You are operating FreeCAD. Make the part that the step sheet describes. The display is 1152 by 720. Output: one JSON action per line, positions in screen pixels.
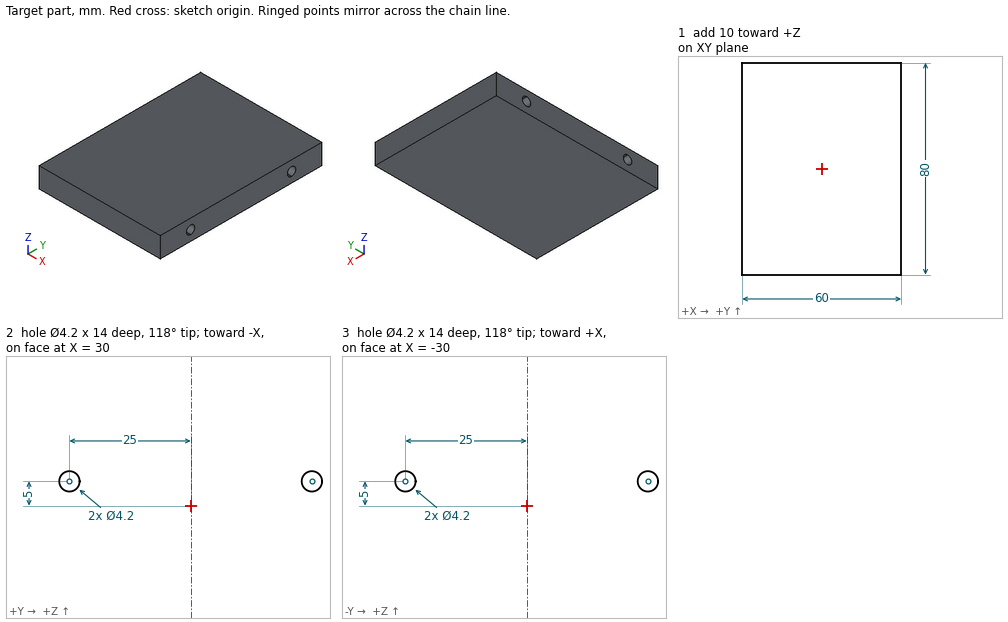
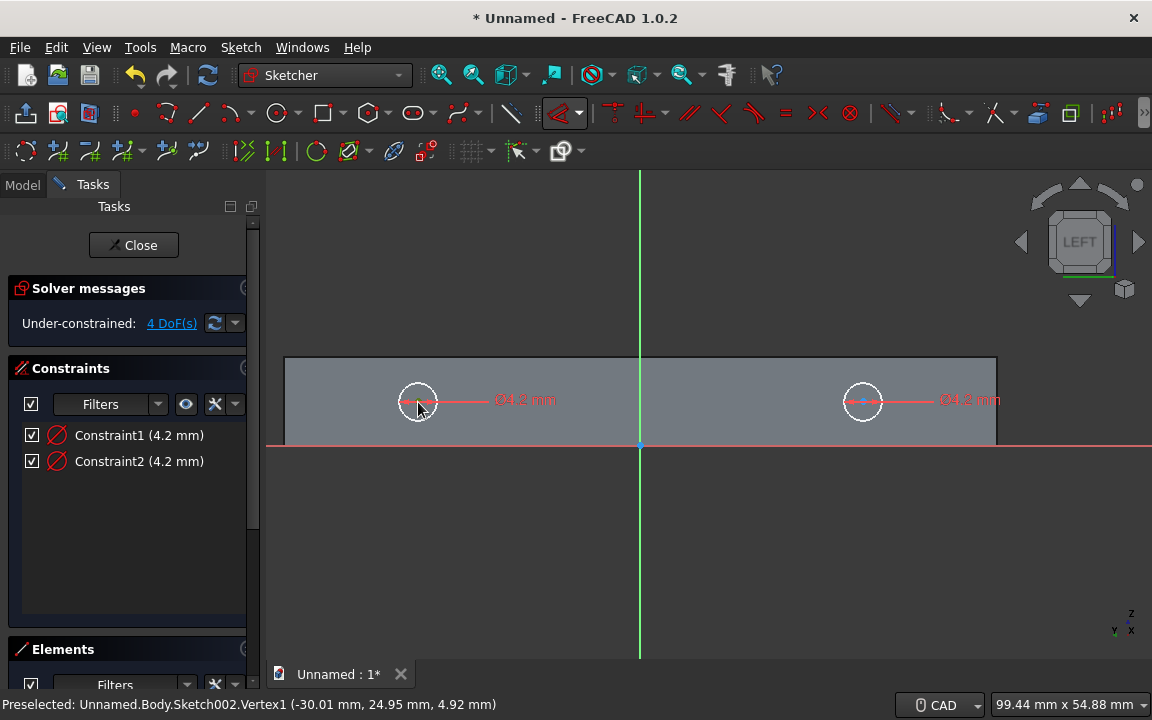
{"action": "left_click", "coordinate": [863, 402]}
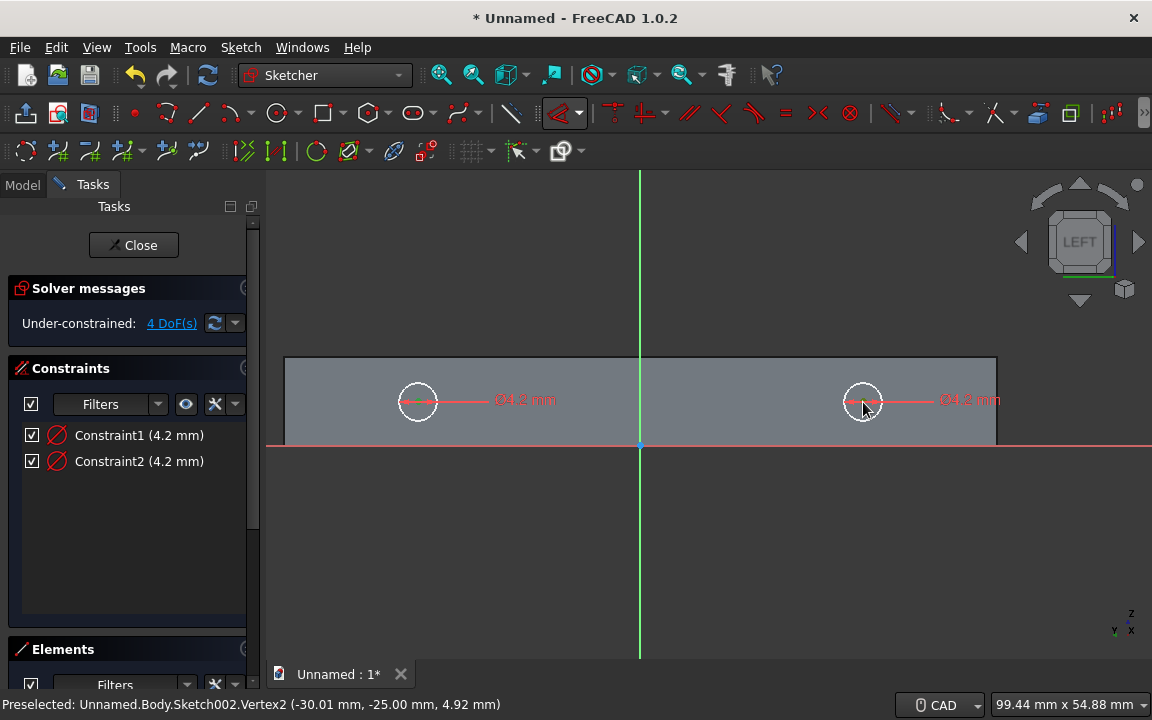
{"action": "left_click", "coordinate": [640, 600]}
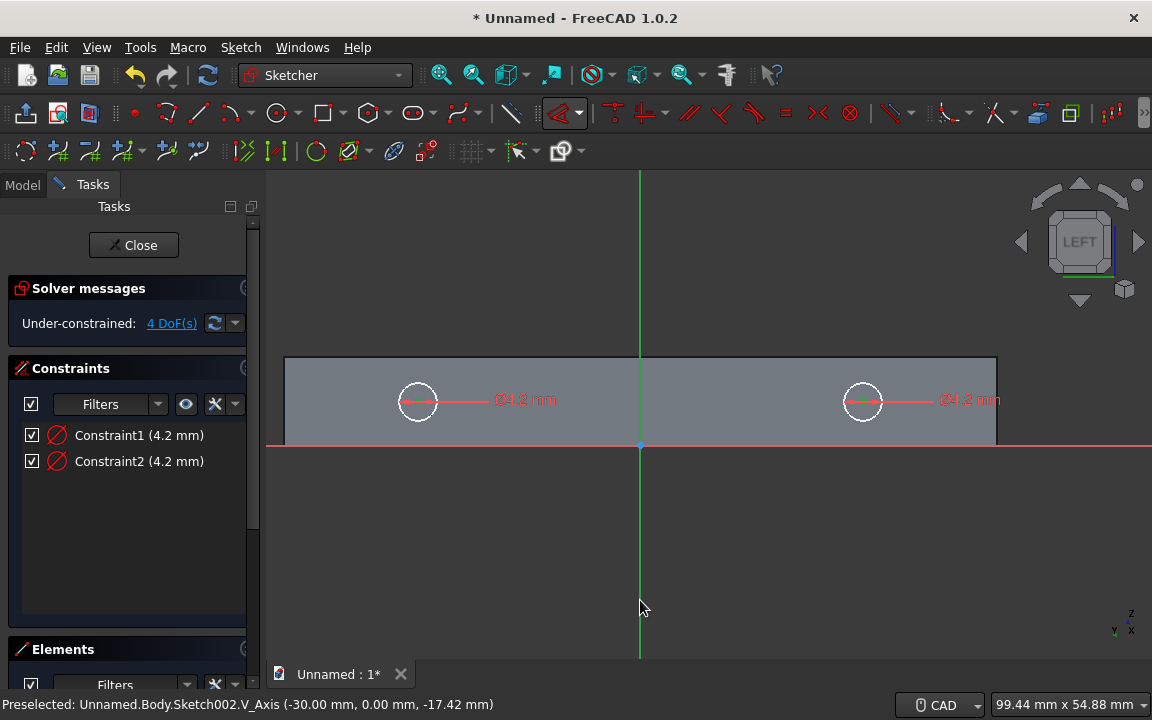
{"action": "left_click", "coordinate": [818, 114]}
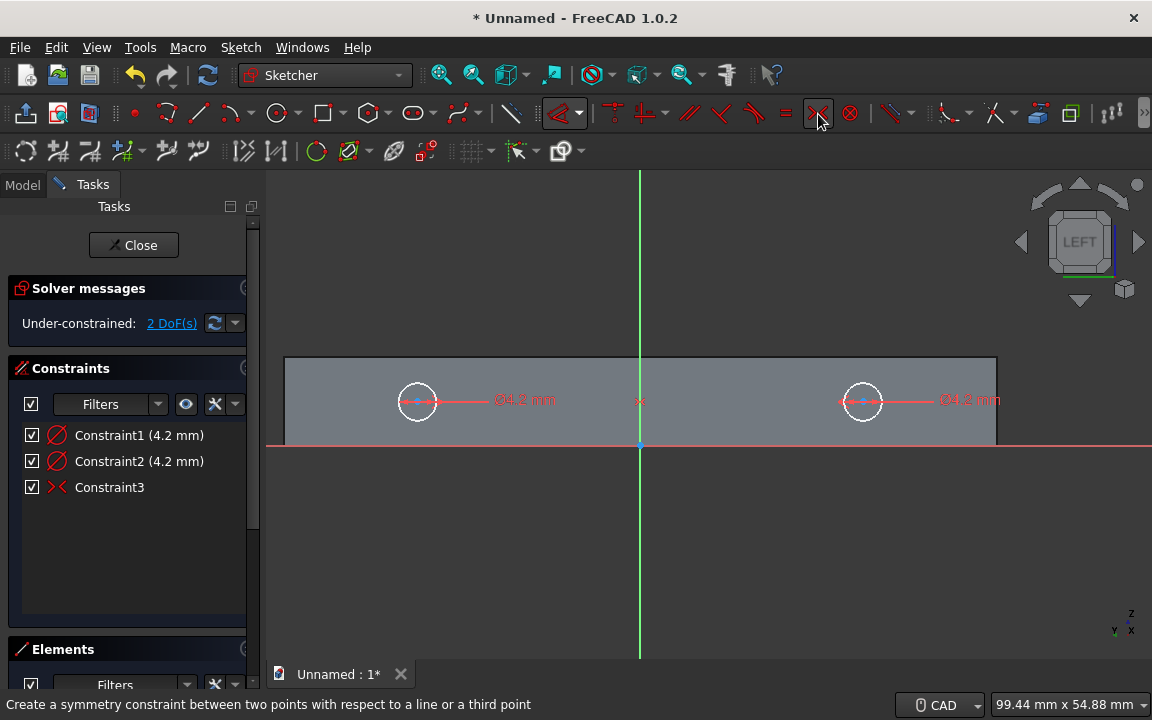
{"action": "left_click", "coordinate": [418, 402]}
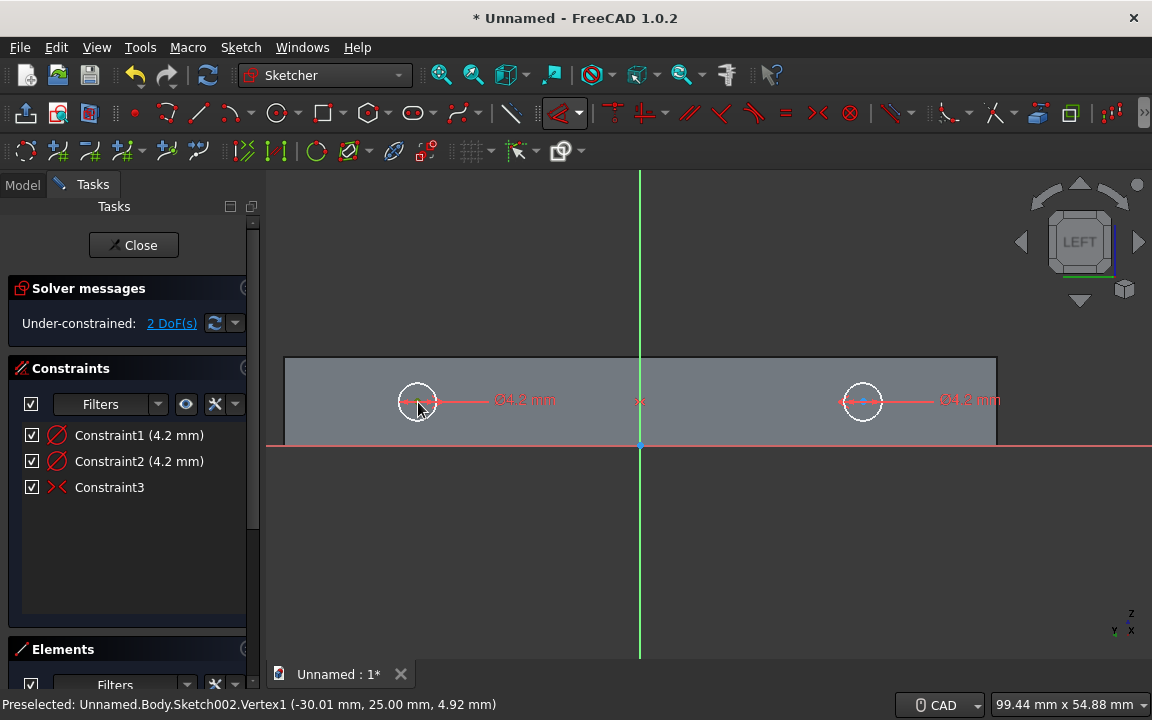
{"action": "left_click", "coordinate": [582, 114]}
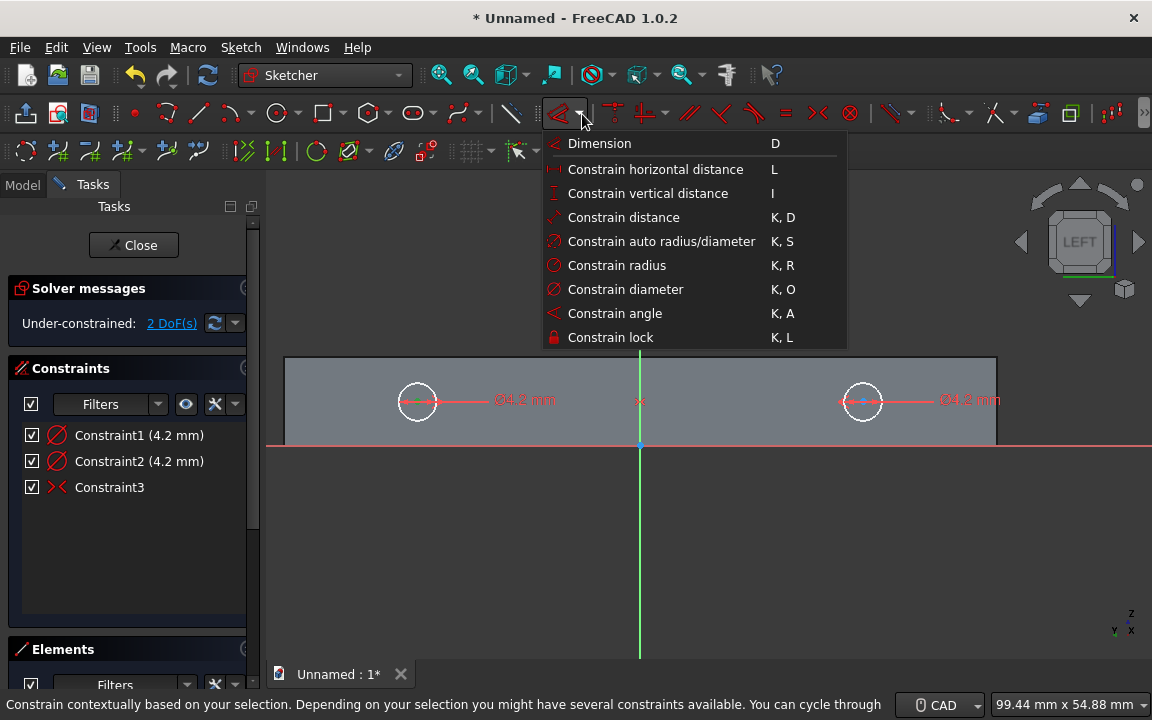
{"action": "left_click", "coordinate": [695, 193]}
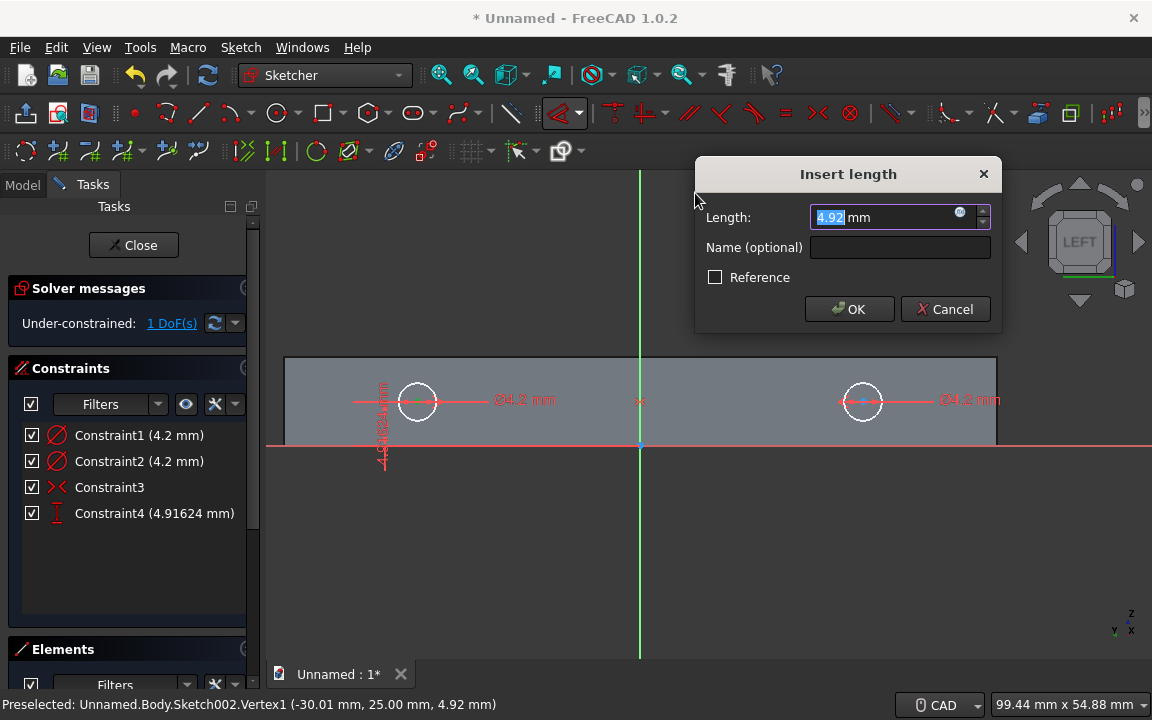
{"action": "type", "text": "5"}
{"action": "key", "text": "Return"}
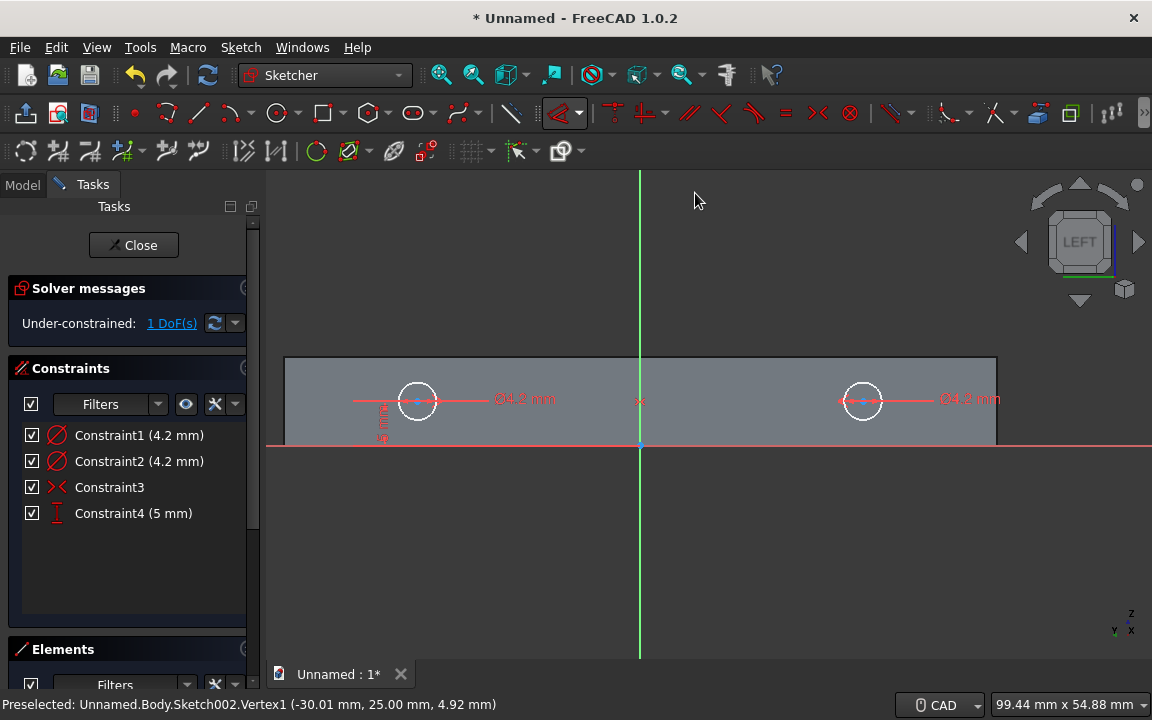
{"action": "left_click", "coordinate": [418, 401]}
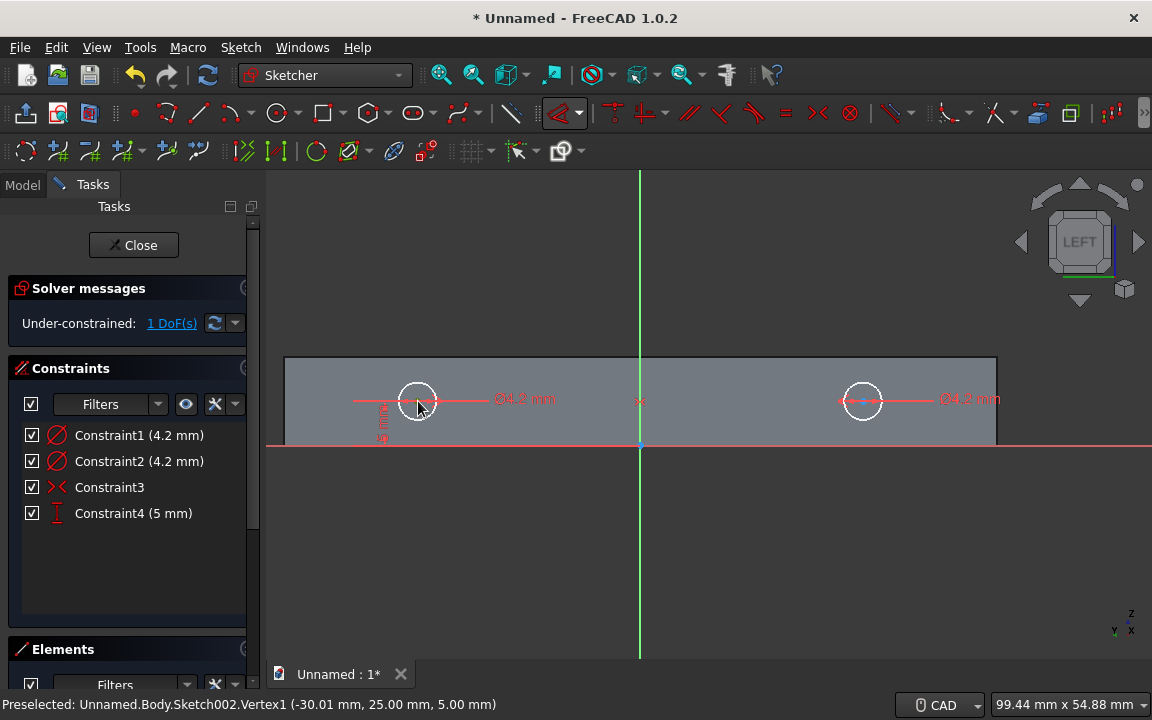
{"action": "left_click", "coordinate": [582, 114]}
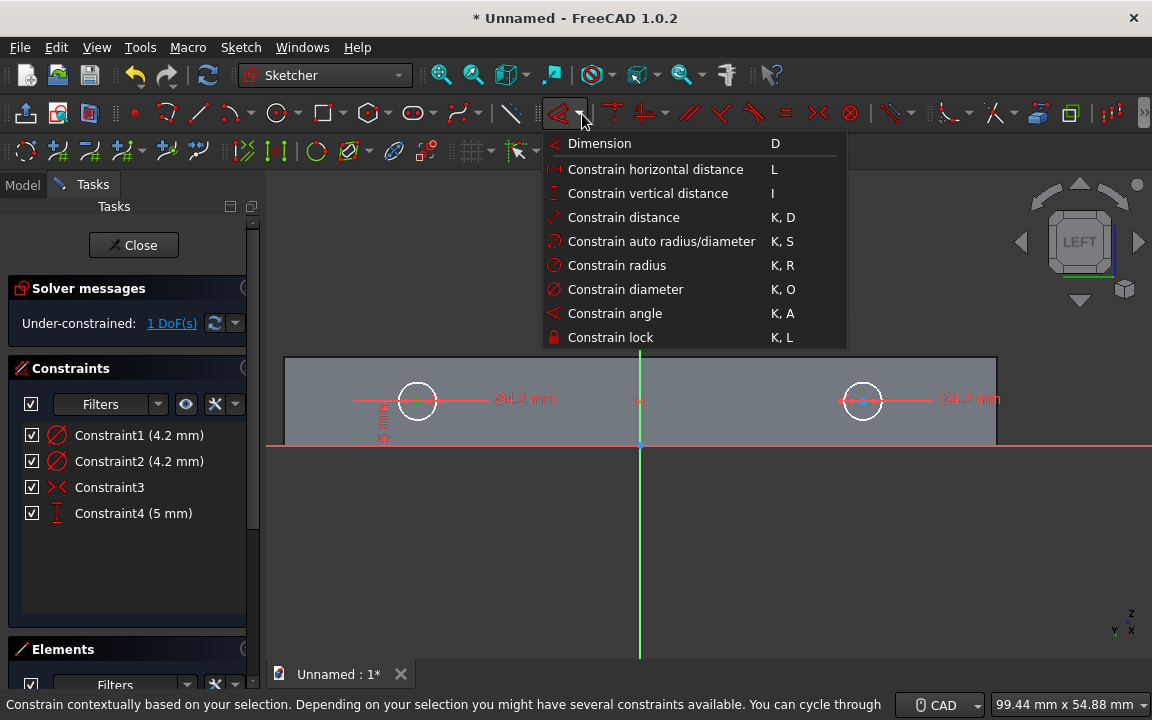
{"action": "left_click", "coordinate": [695, 169]}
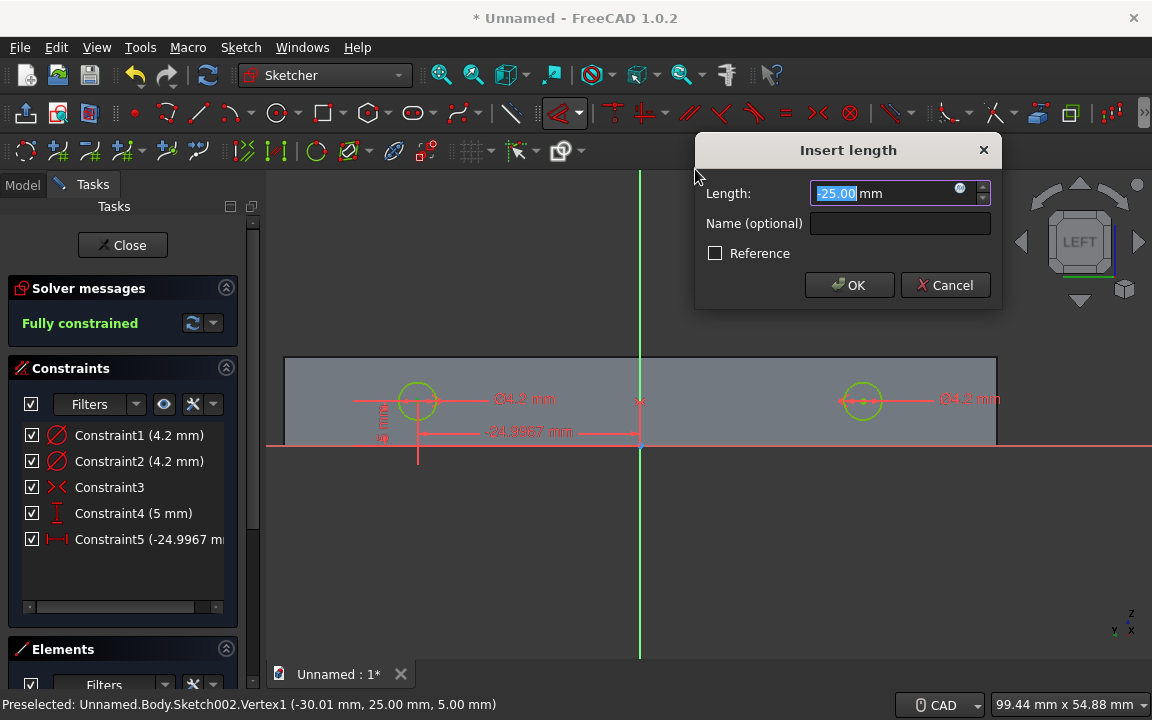
{"action": "type", "text": "-25"}
{"action": "key", "text": "Return"}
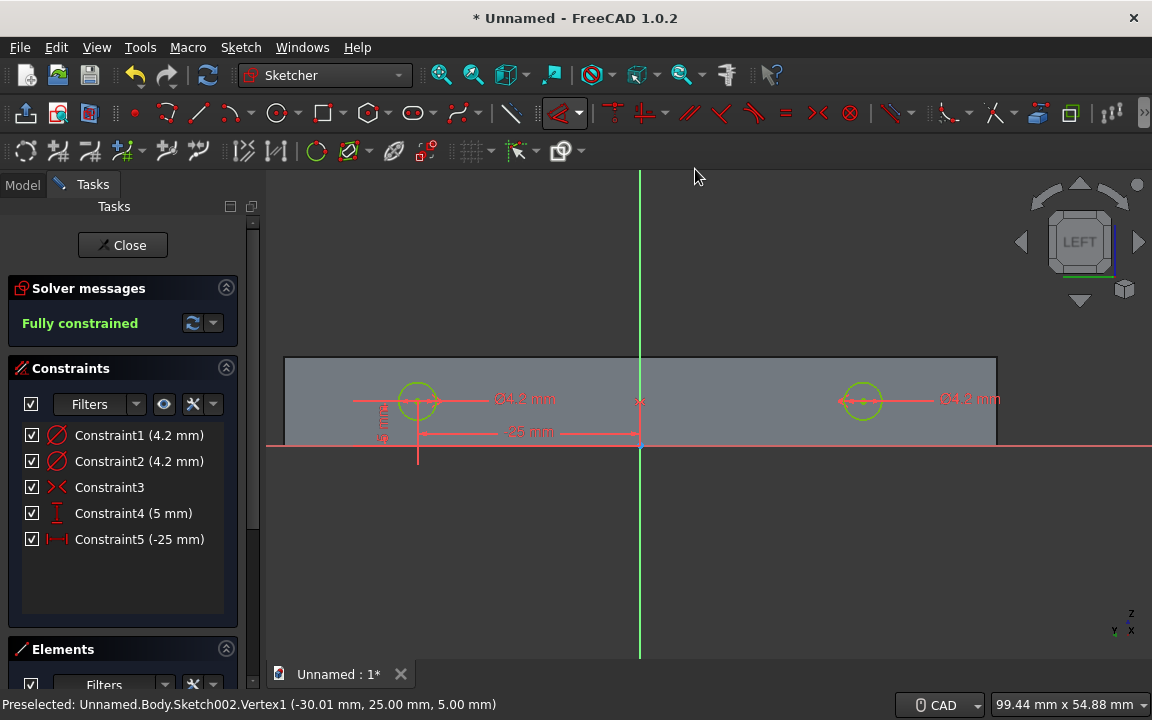
{"action": "left_click", "coordinate": [123, 245]}